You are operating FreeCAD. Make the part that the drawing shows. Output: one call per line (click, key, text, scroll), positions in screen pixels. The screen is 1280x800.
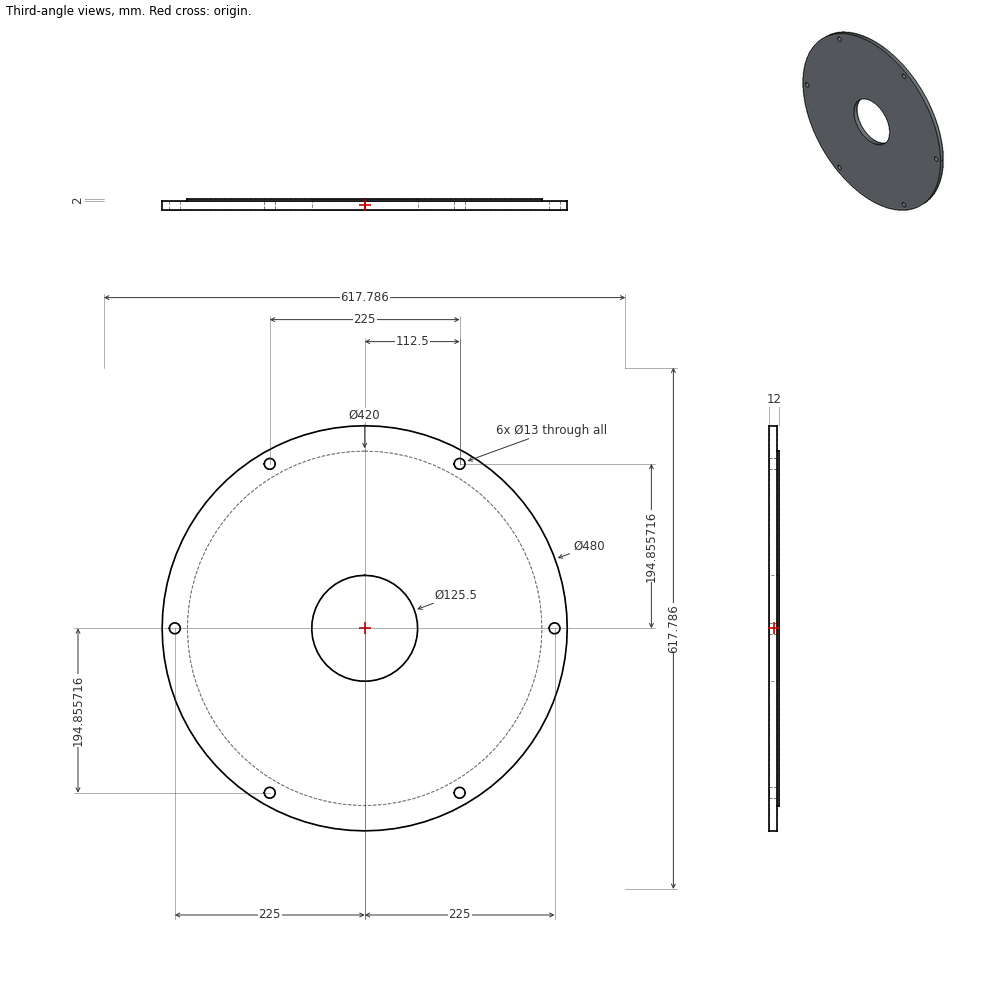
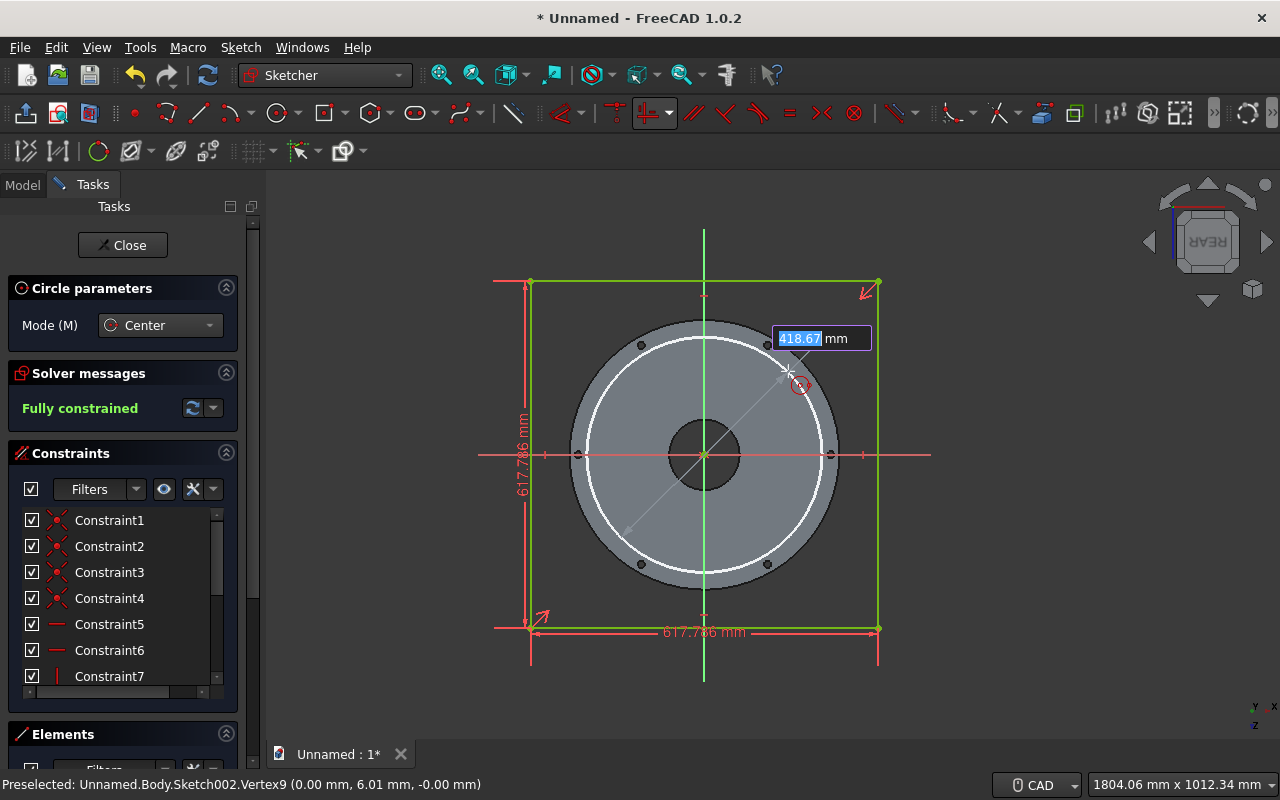
text(420)
key(Return)
key(Escape)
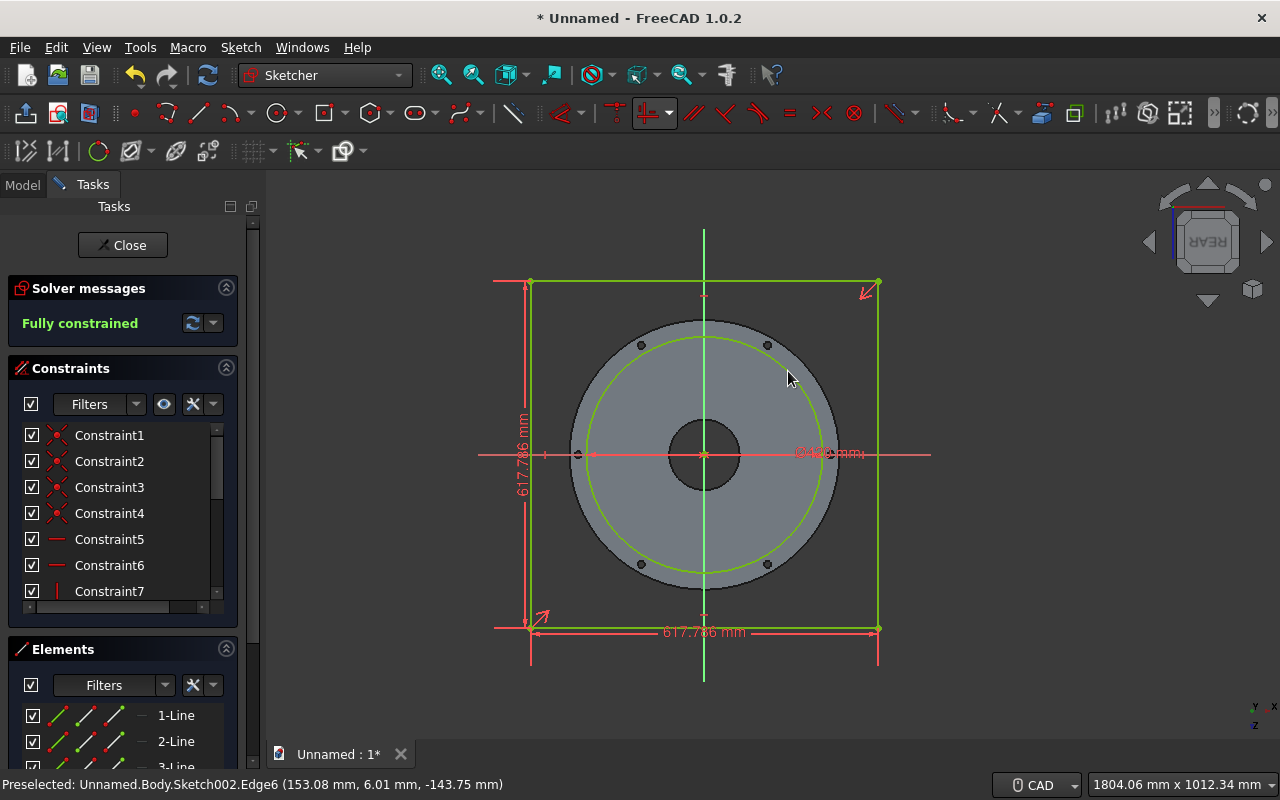
click(123, 245)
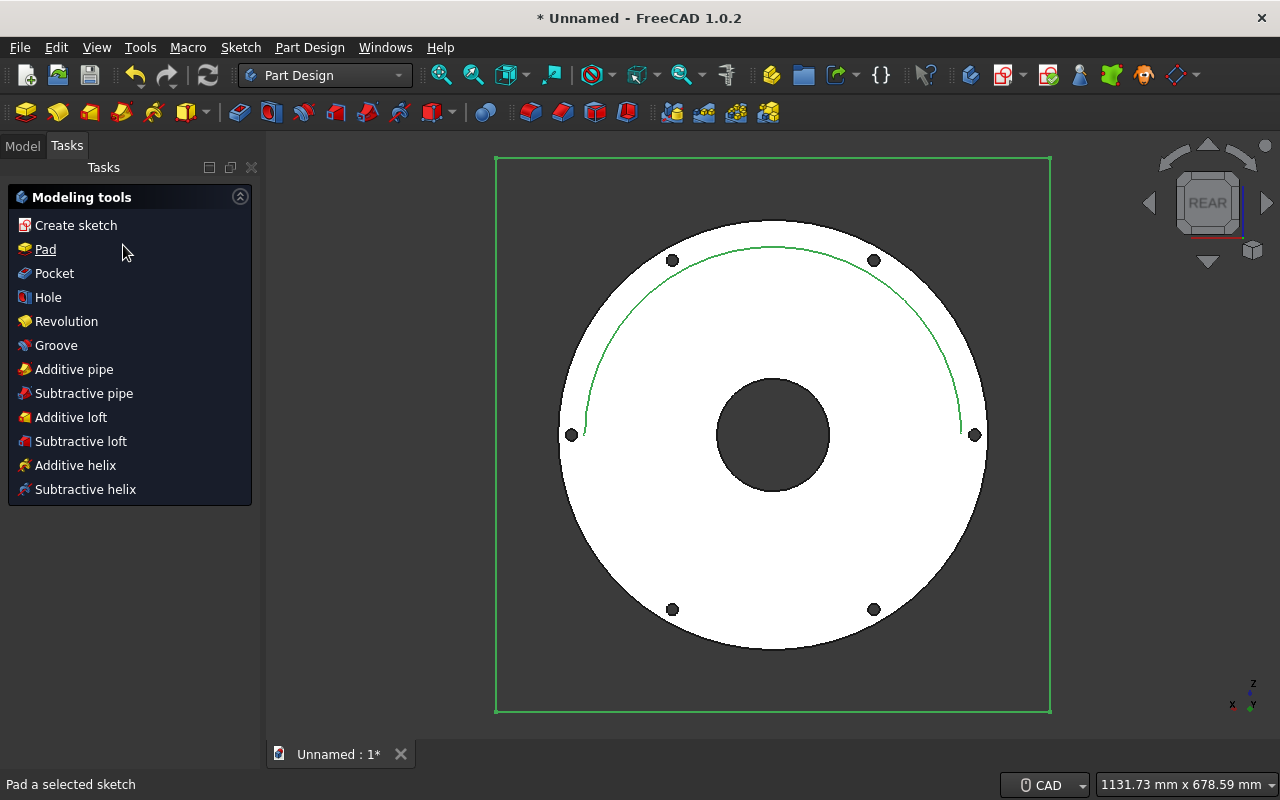
click(240, 112)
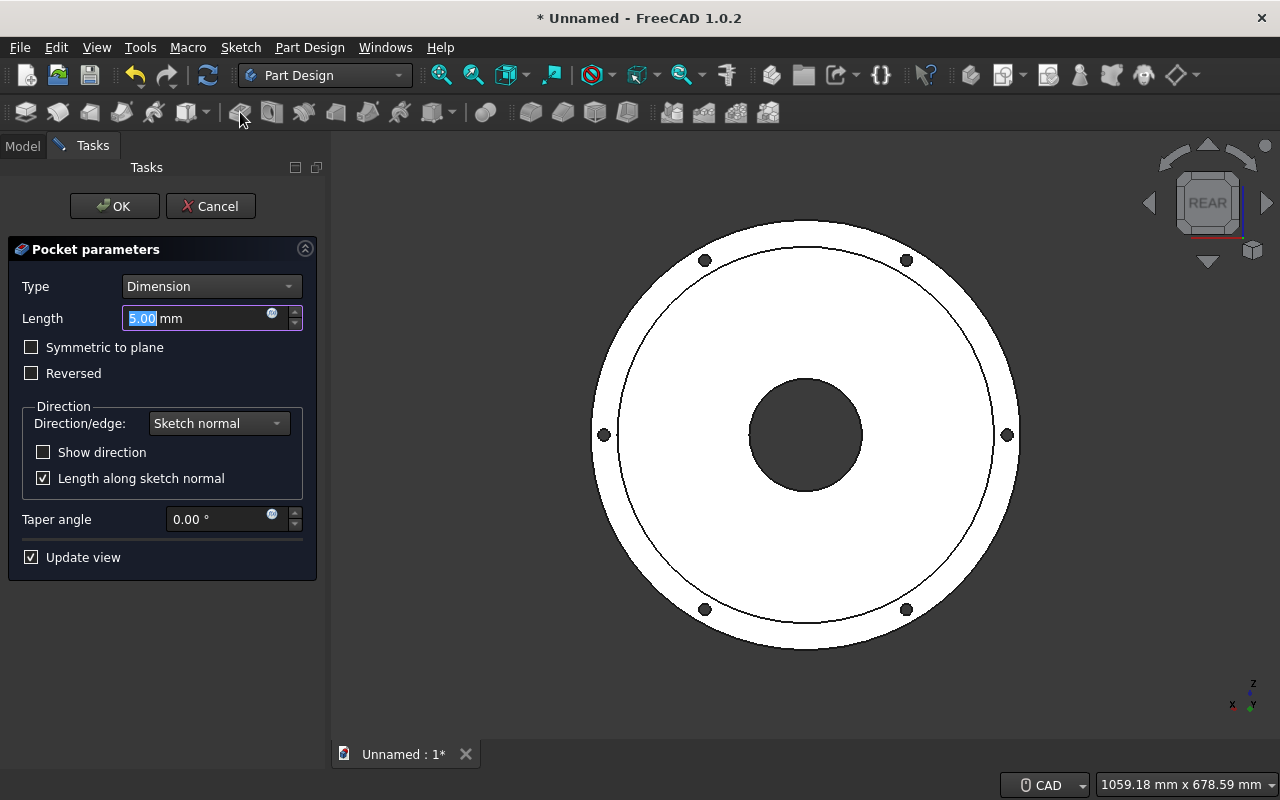
text(2)
key(Tab)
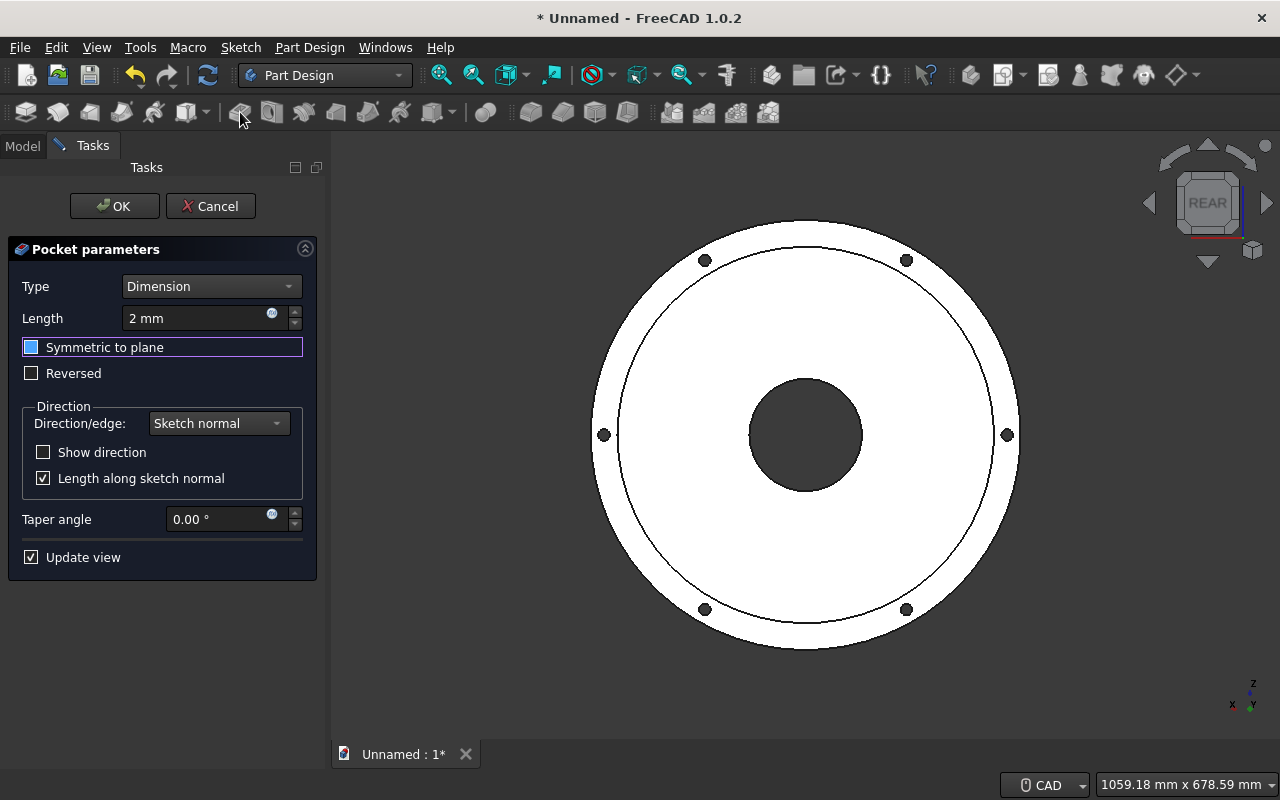
click(115, 206)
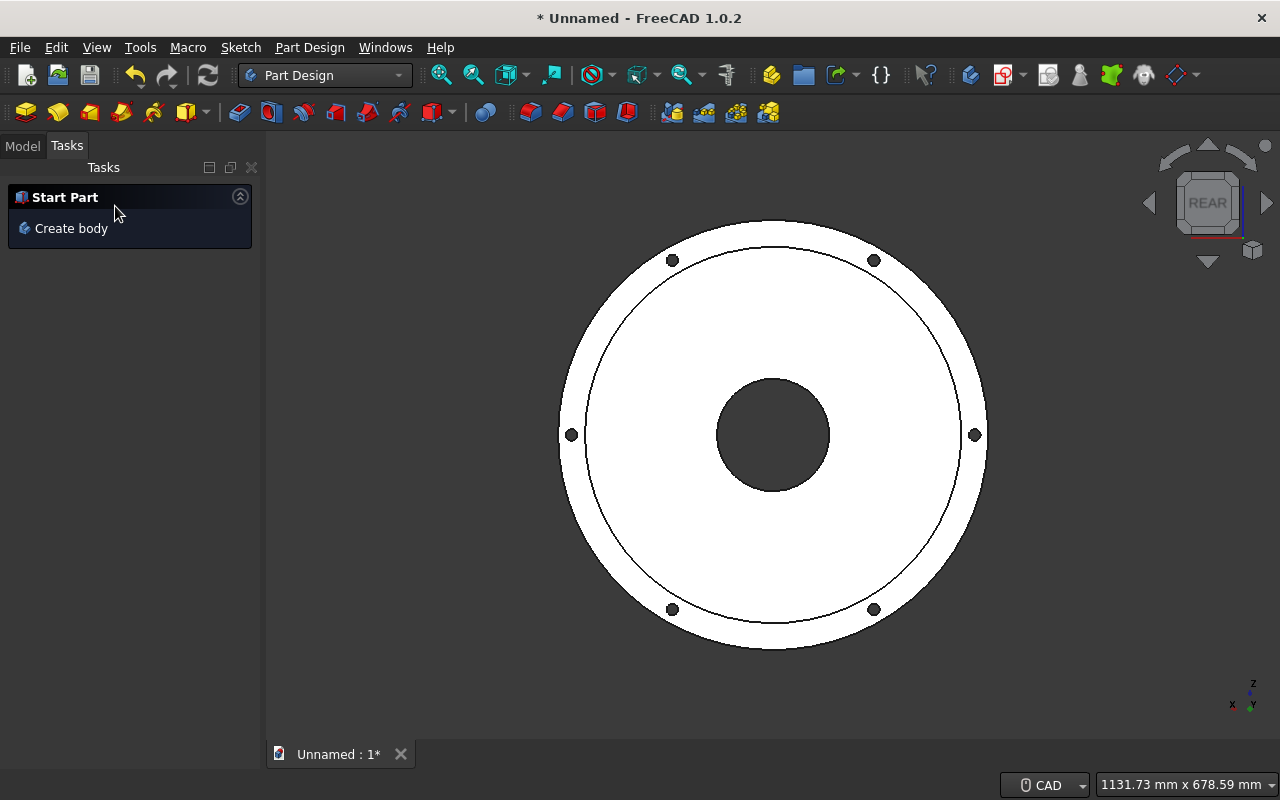
key(0)